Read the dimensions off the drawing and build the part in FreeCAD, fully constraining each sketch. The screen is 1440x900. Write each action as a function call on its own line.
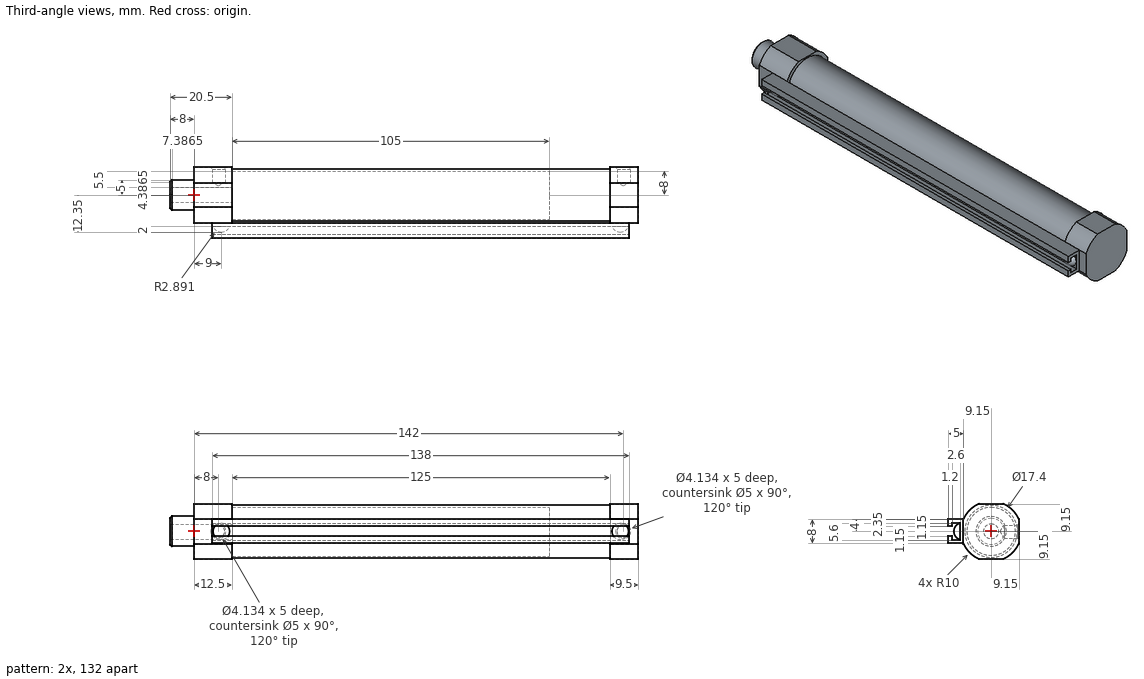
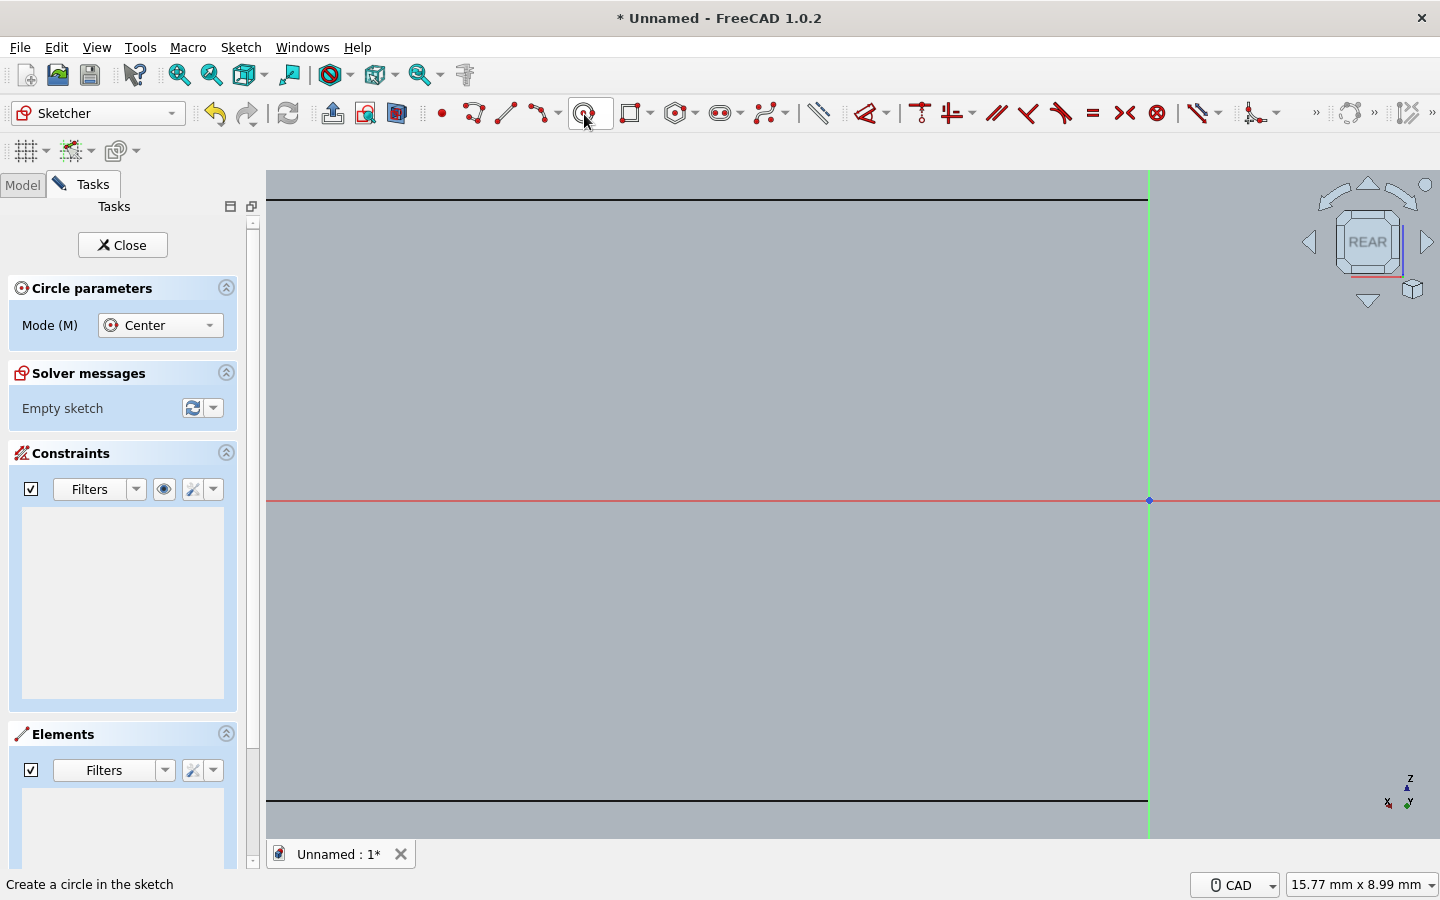
click(554, 501)
click(662, 392)
key(Escape)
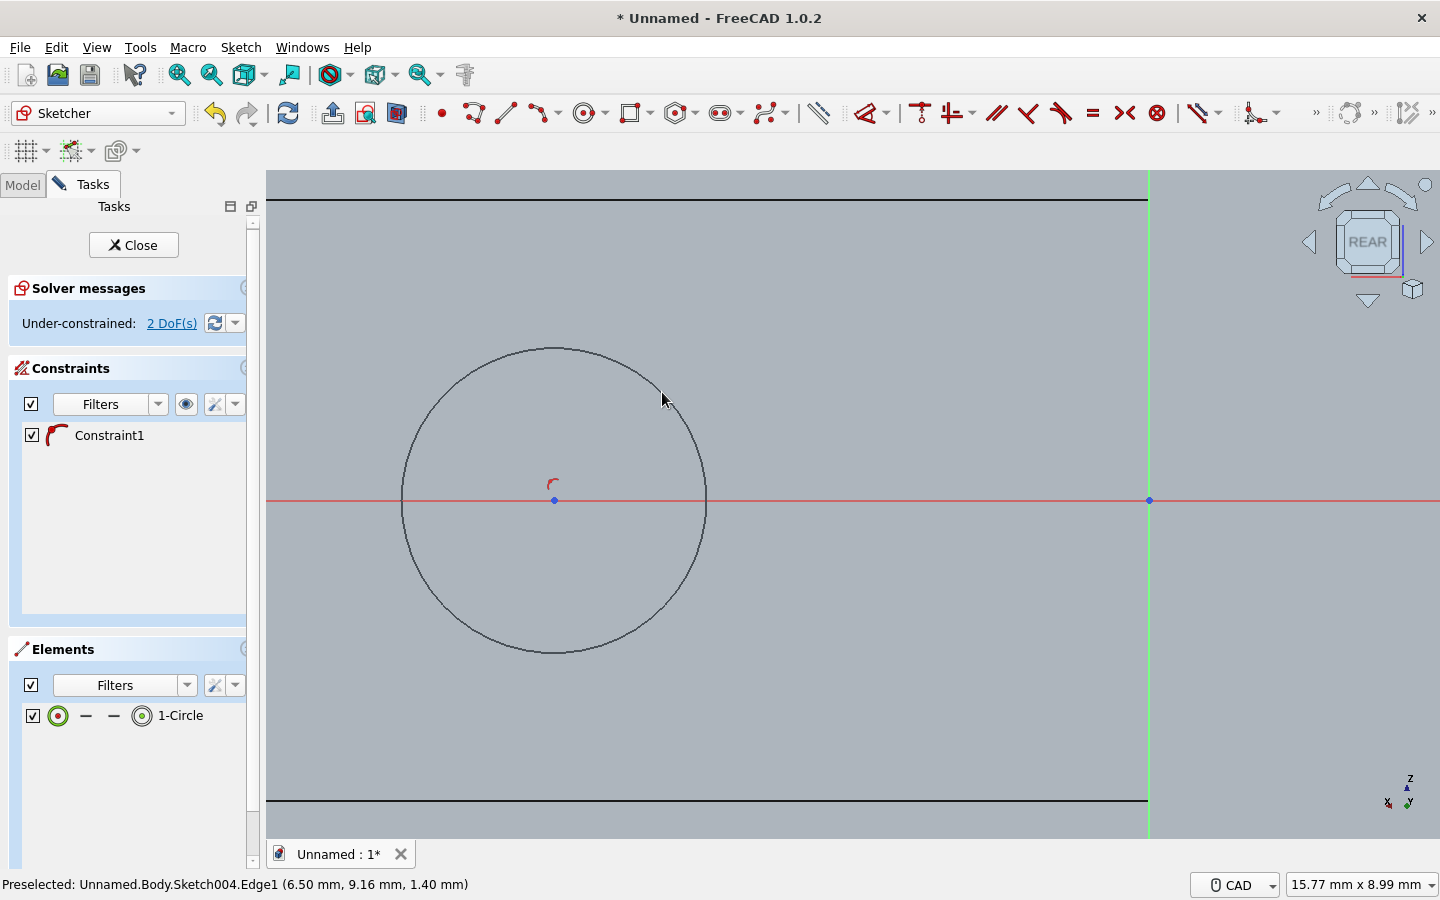
click(866, 114)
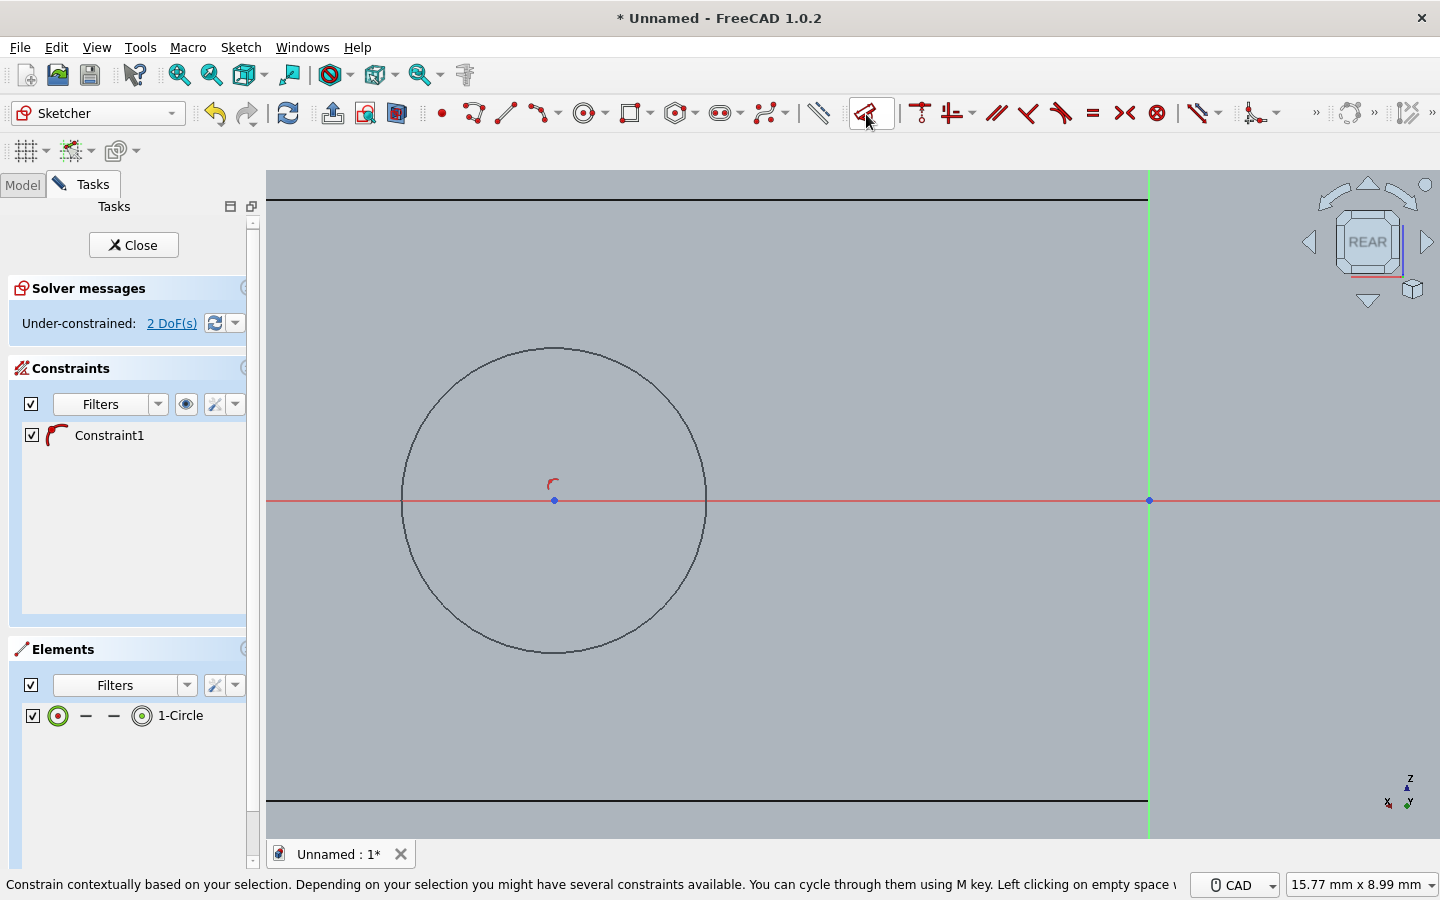
click(662, 393)
click(685, 370)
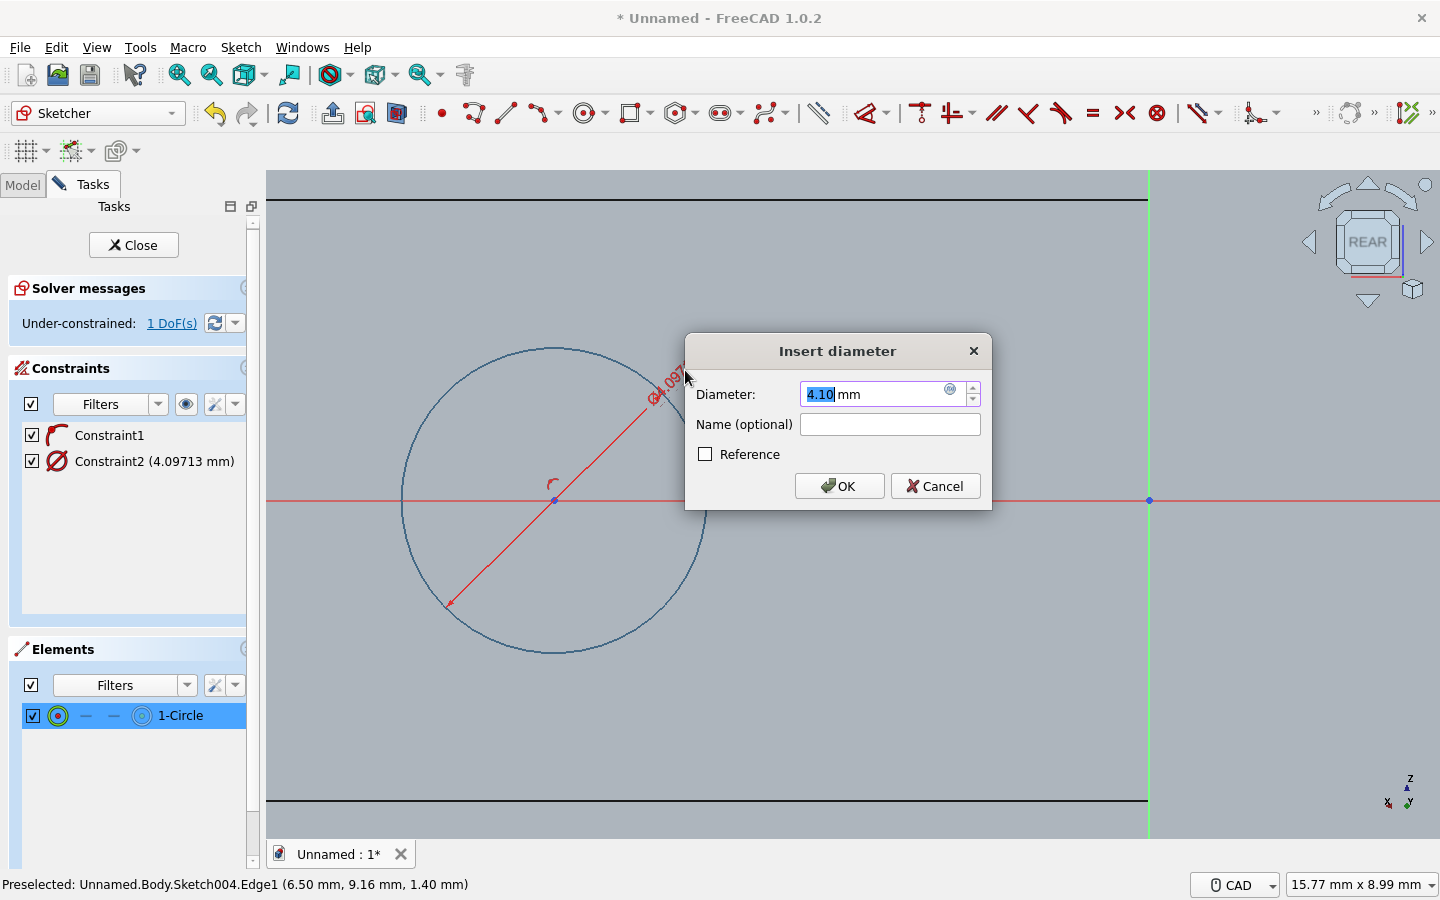
text(4.134)
key(Return)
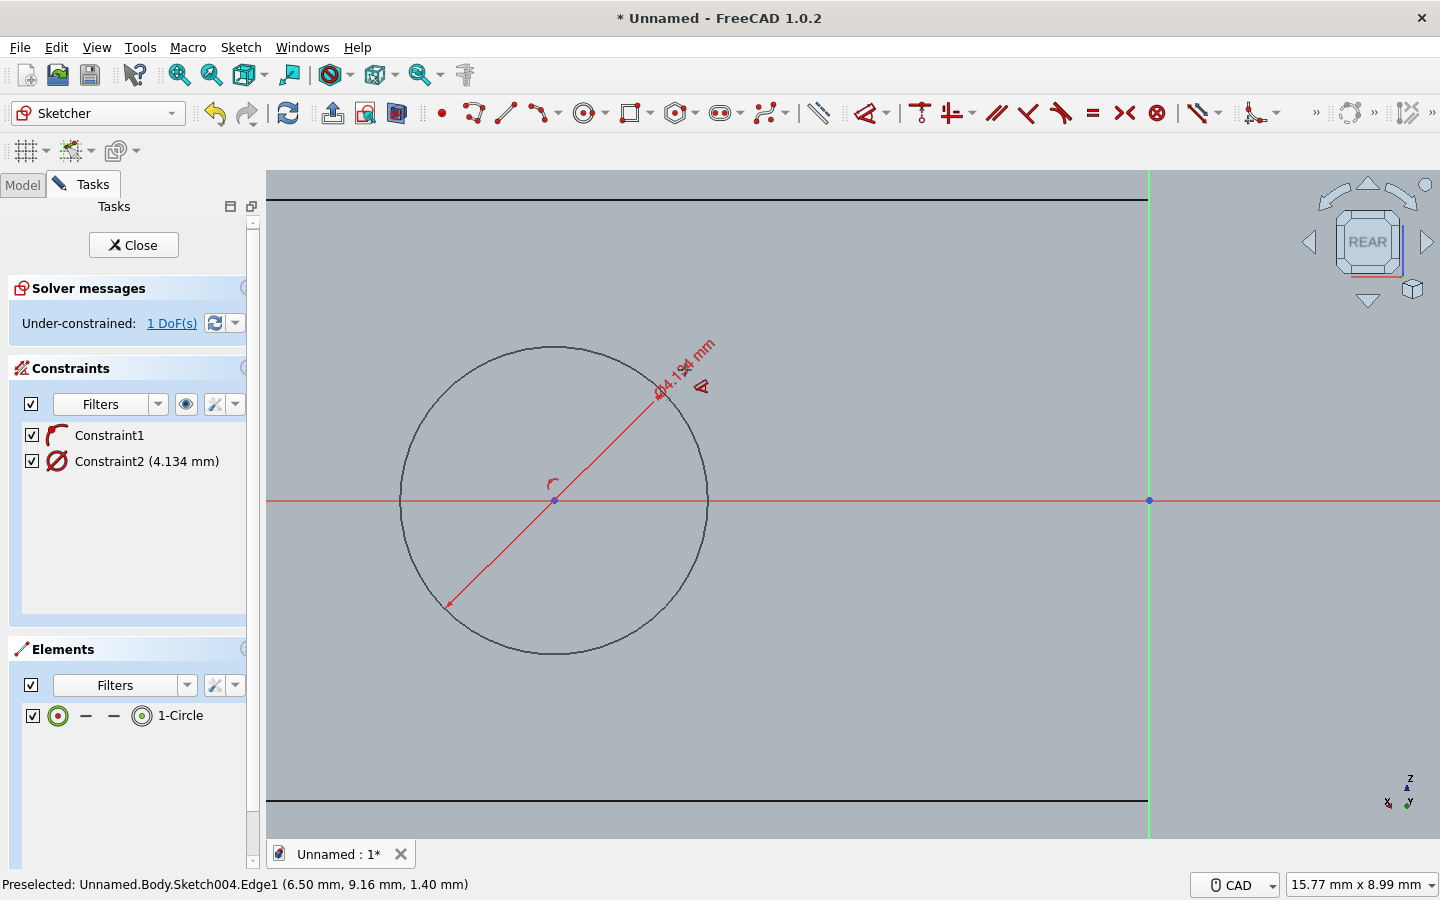
click(554, 501)
click(852, 535)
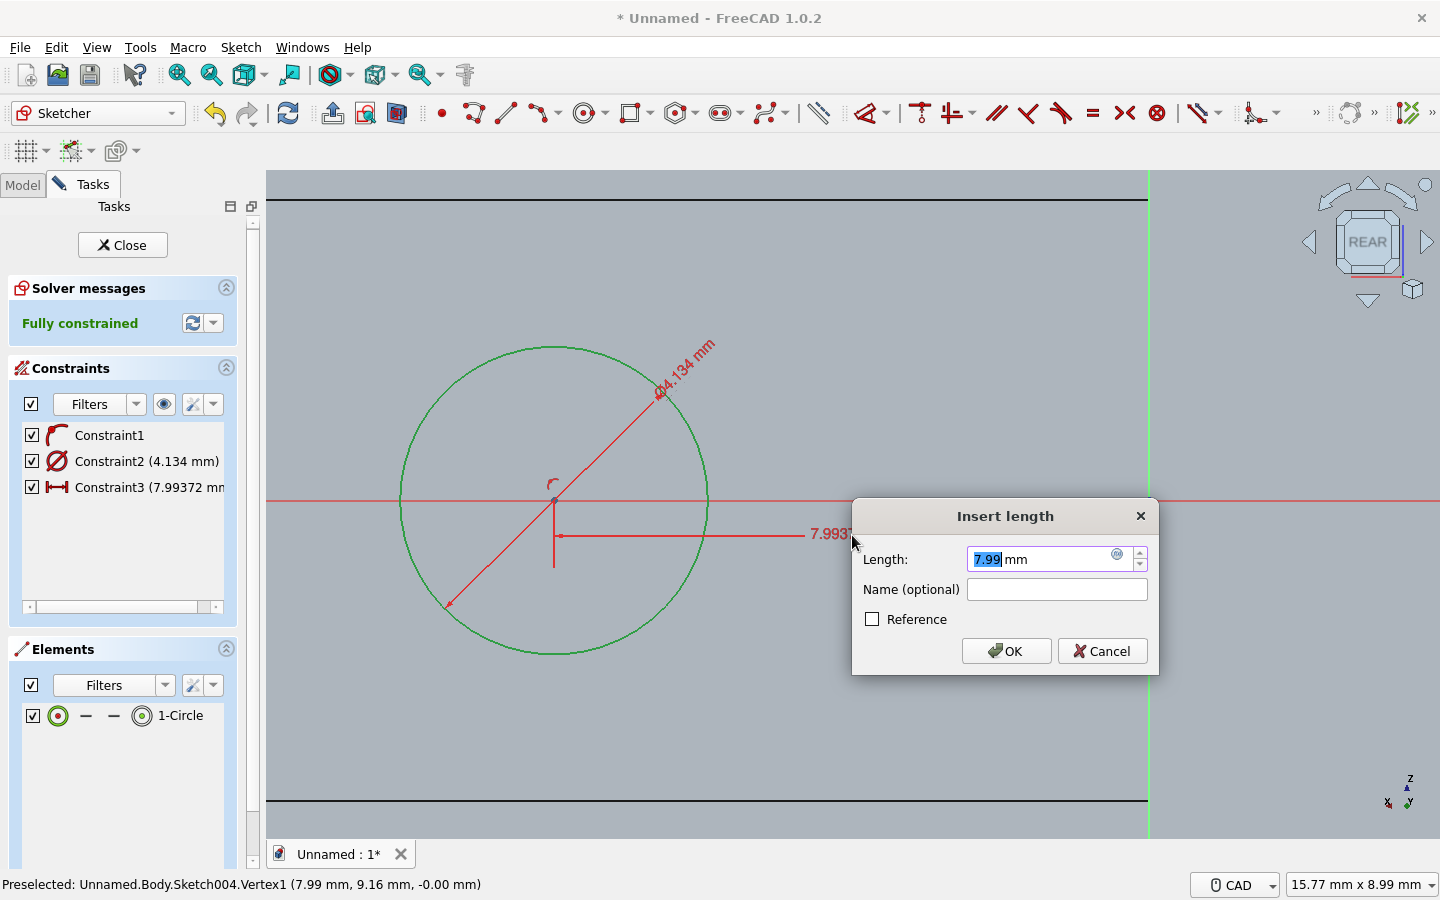
text(8)
key(Return)
key(Escape)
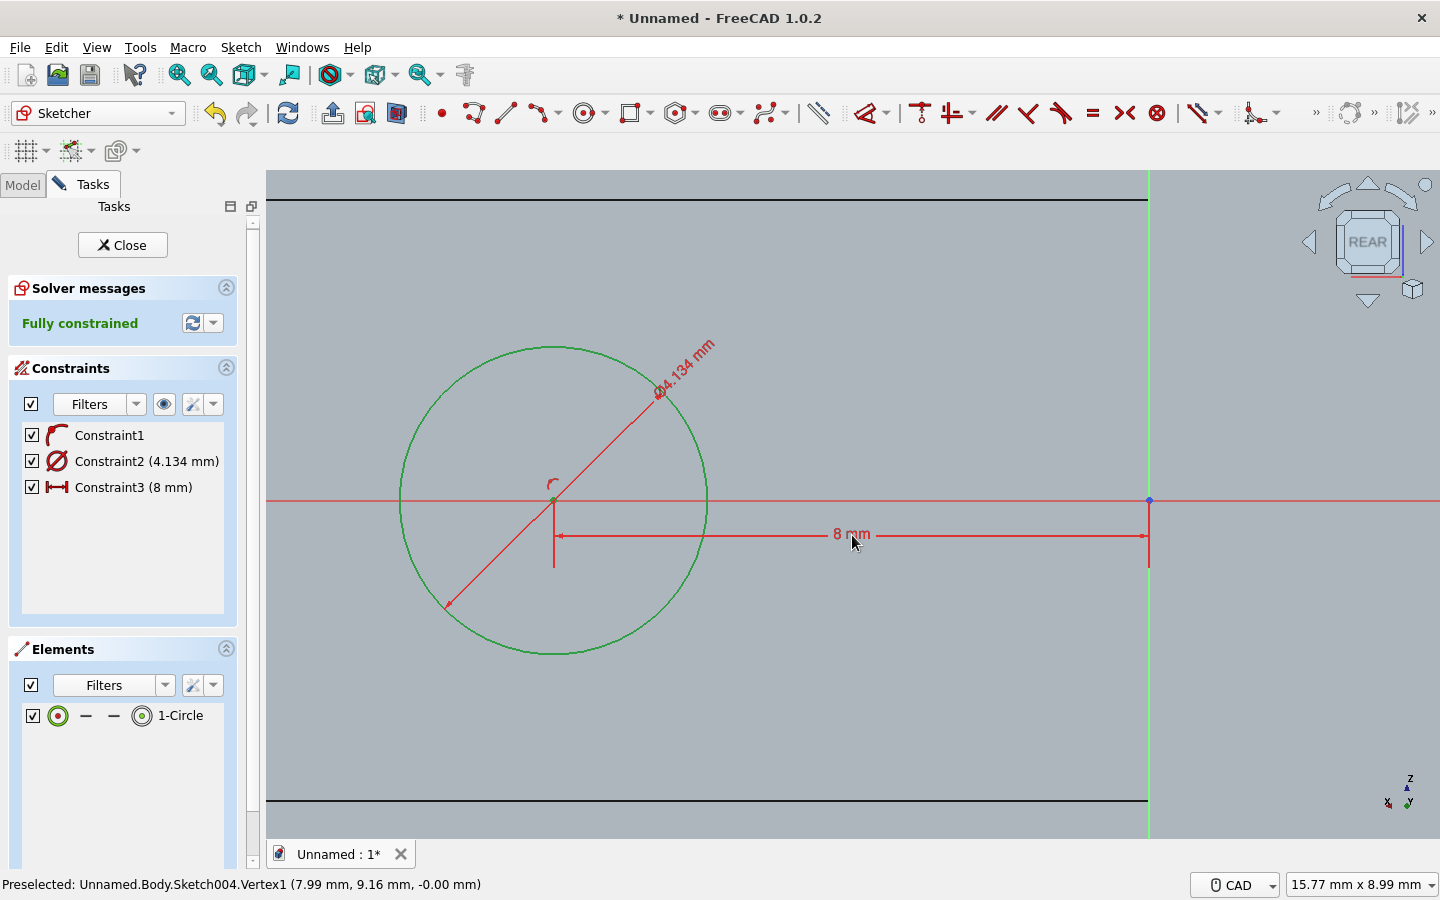
click(123, 245)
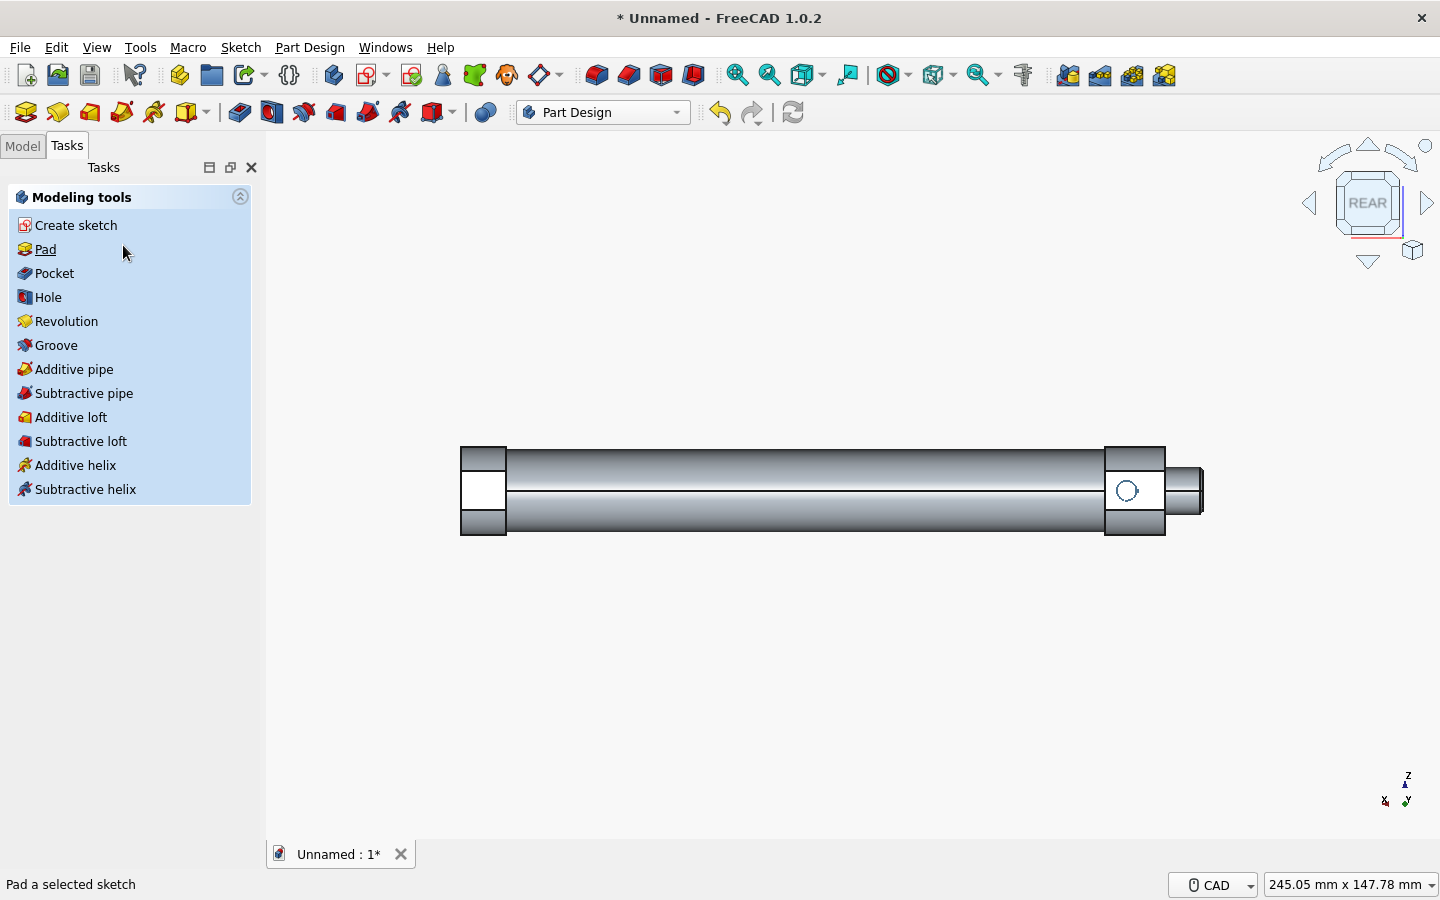
click(272, 112)